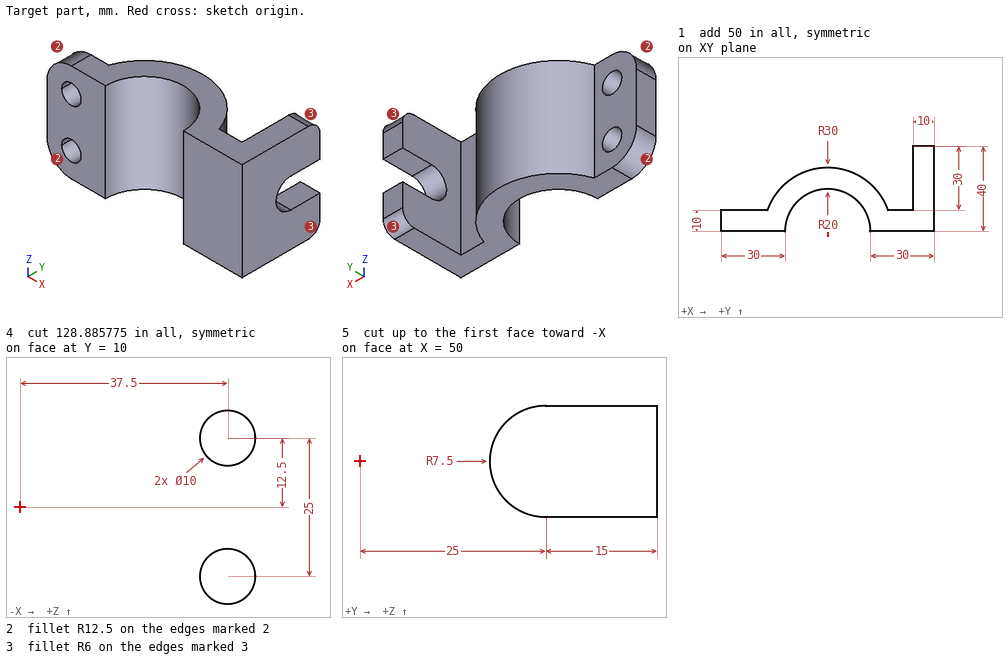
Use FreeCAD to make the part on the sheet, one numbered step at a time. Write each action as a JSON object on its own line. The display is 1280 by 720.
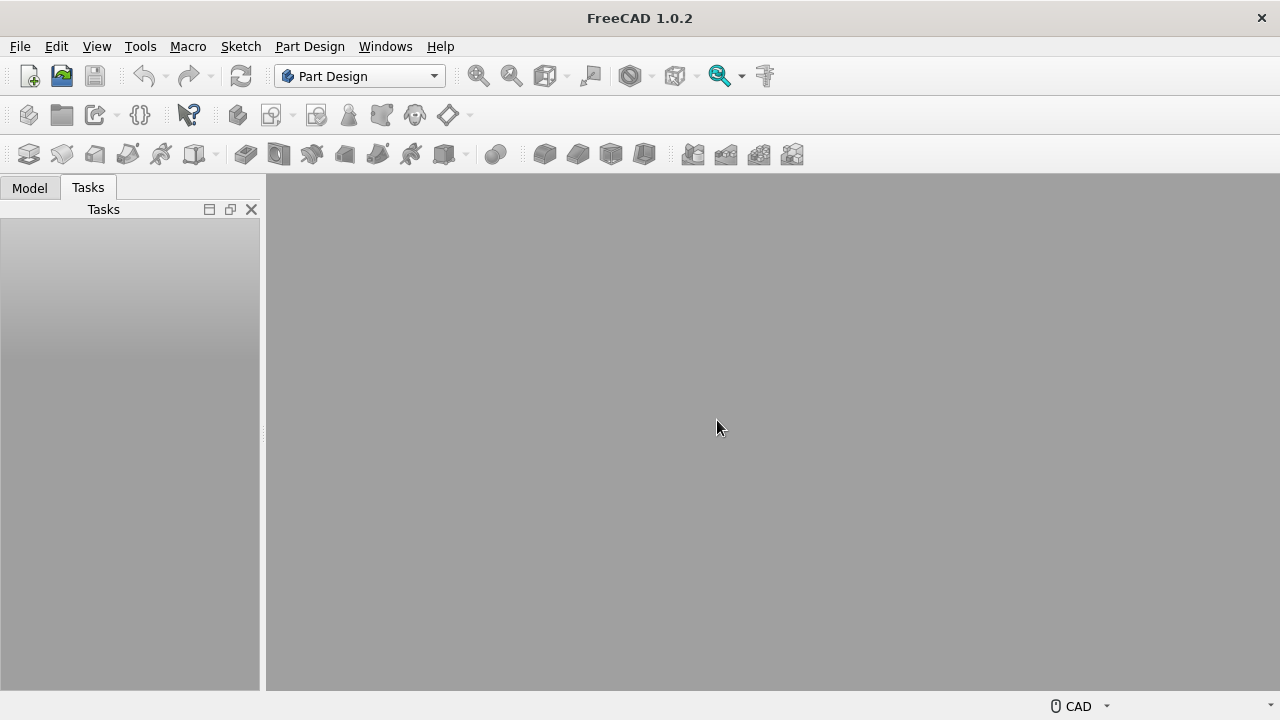
{"action": "left_click", "coordinate": [29, 76]}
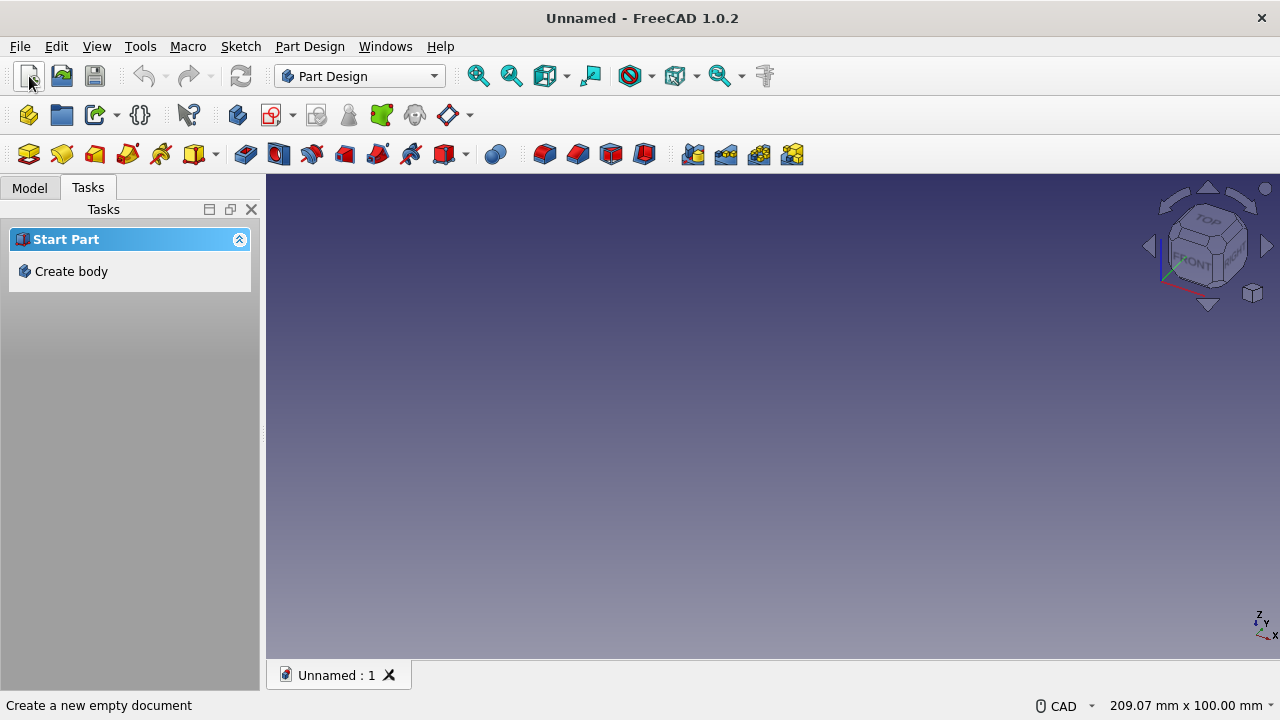
{"action": "left_click", "coordinate": [270, 116]}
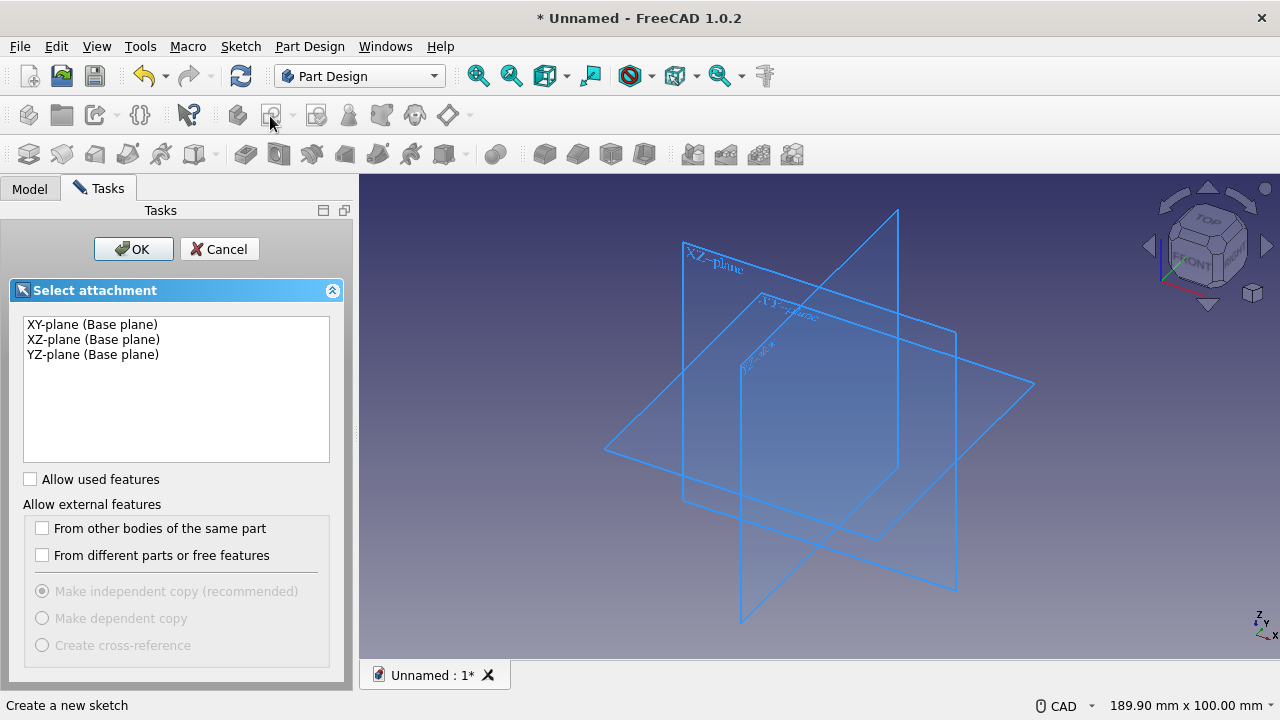
{"action": "left_click", "coordinate": [84, 324]}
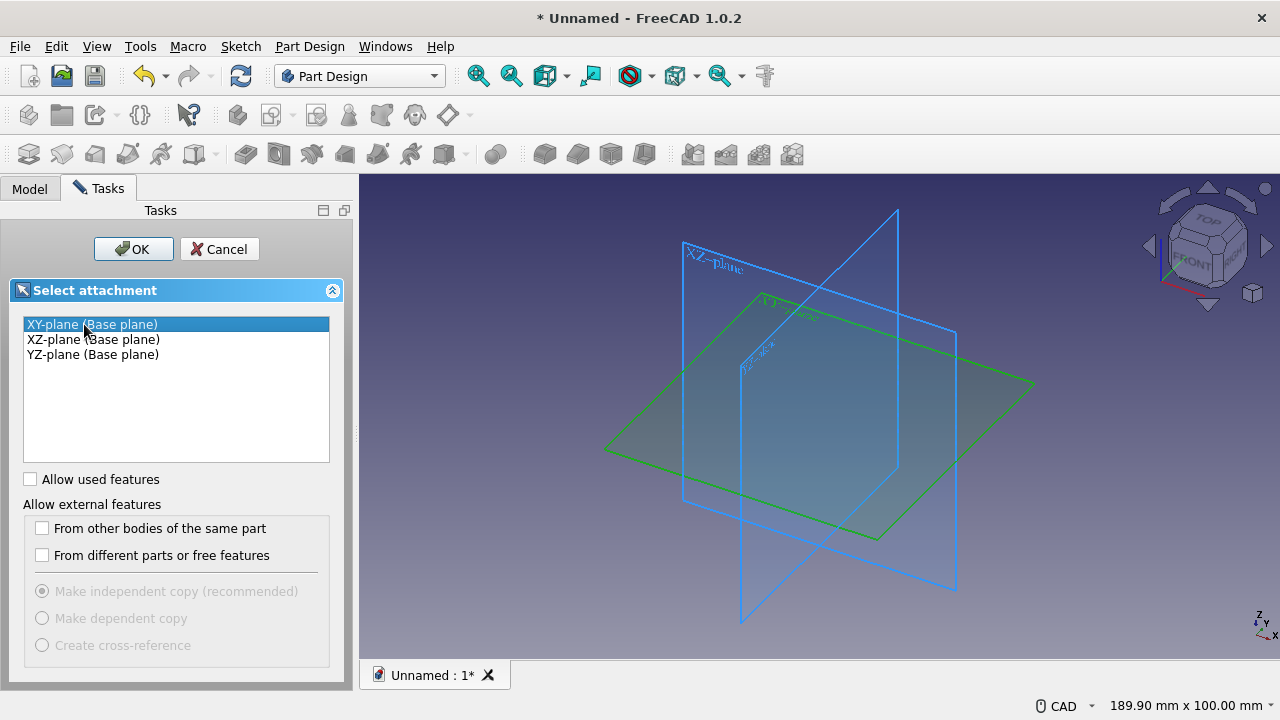
{"action": "left_click", "coordinate": [134, 249]}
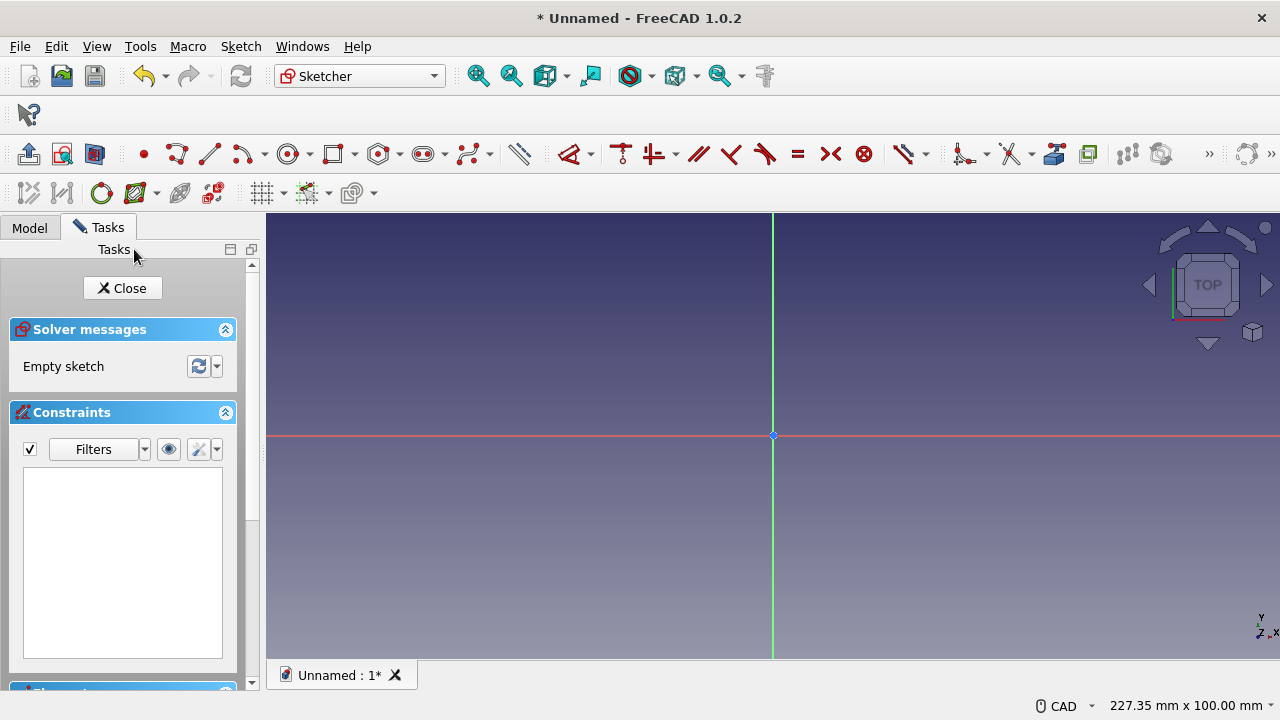
{"action": "scroll", "coordinate": [395, 631], "scroll_direction": "down", "scroll_amount": 1}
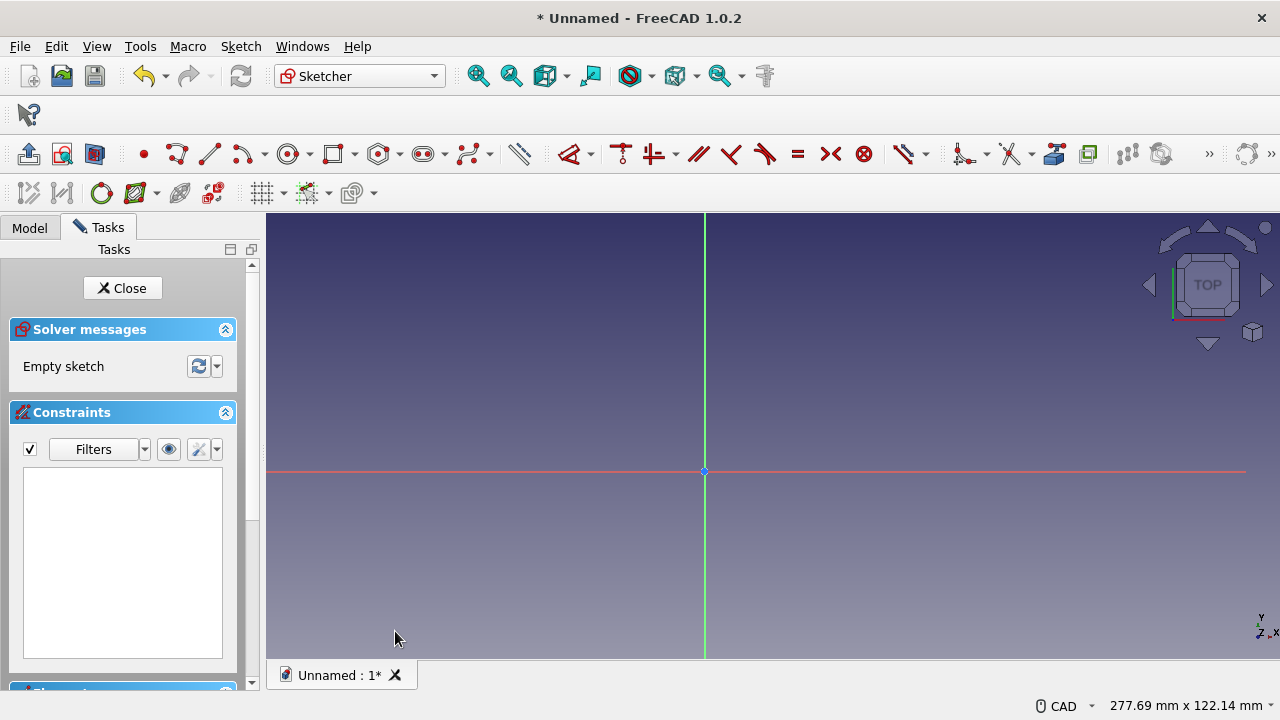
{"action": "scroll", "coordinate": [705, 322], "scroll_direction": "up", "scroll_amount": 2}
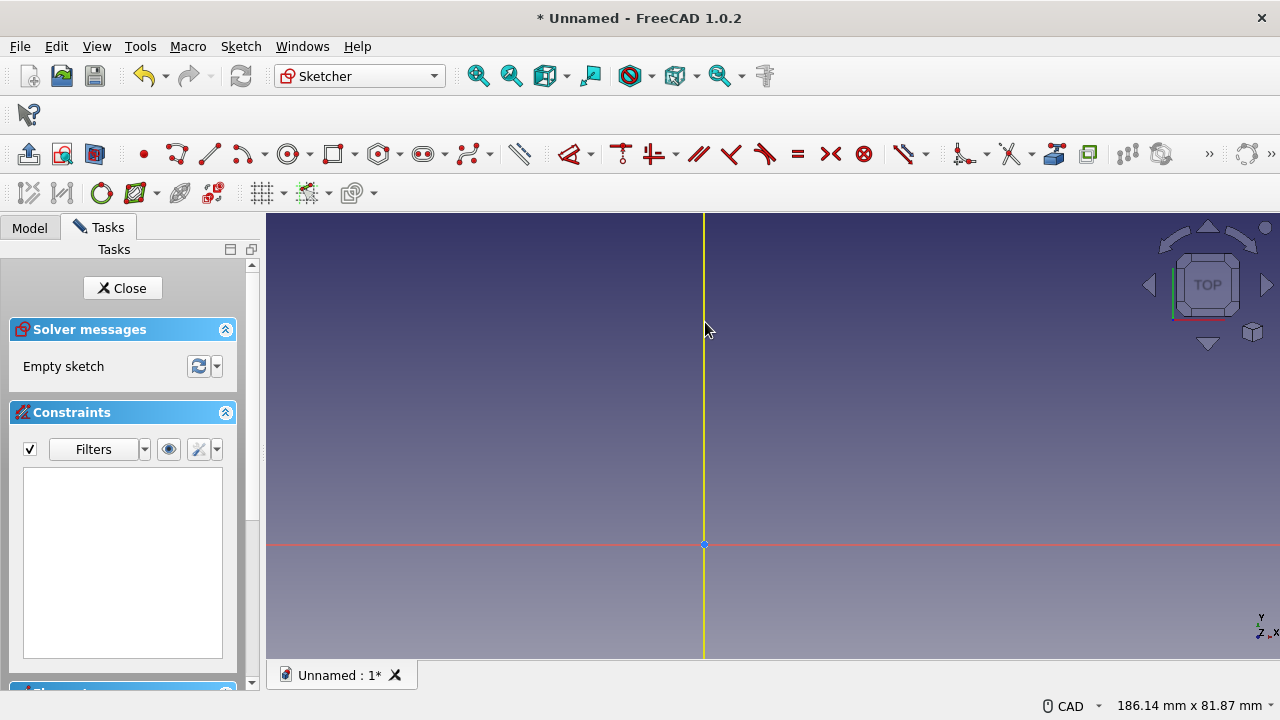
{"action": "left_click", "coordinate": [177, 154]}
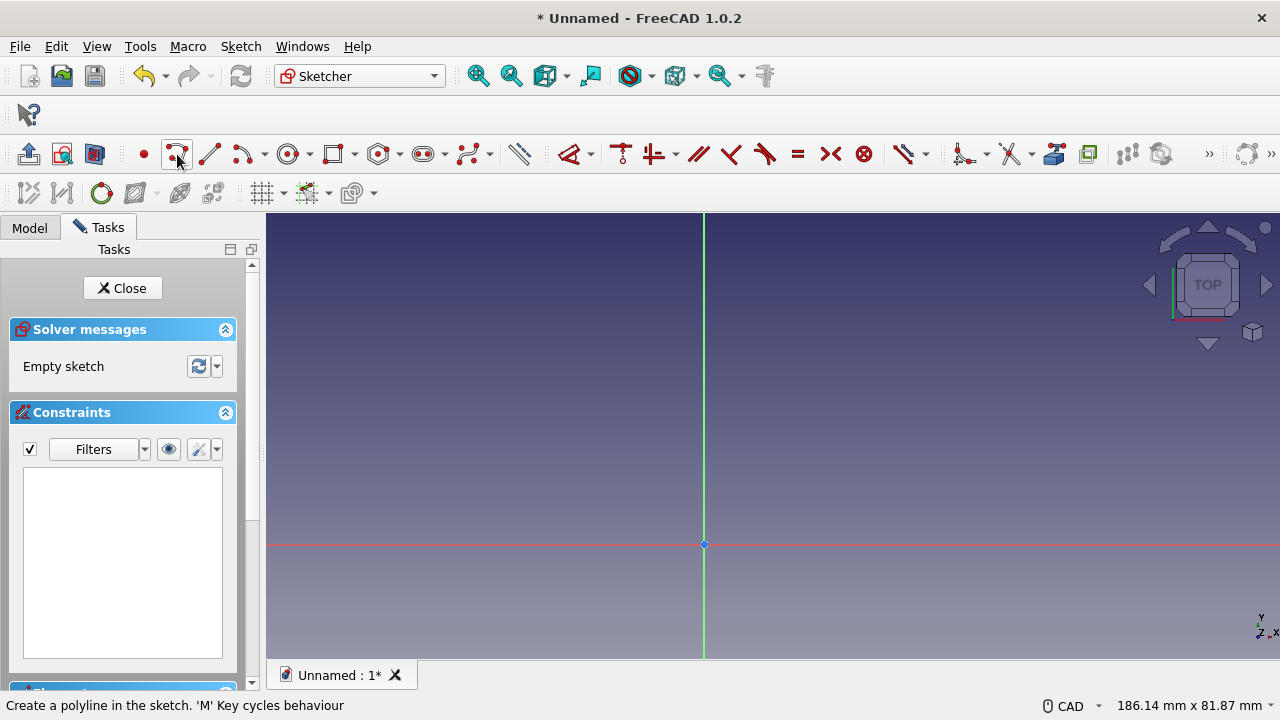
{"action": "left_click", "coordinate": [550, 490]}
{"action": "left_click", "coordinate": [432, 490]}
{"action": "left_click", "coordinate": [432, 545]}
{"action": "left_click", "coordinate": [595, 536]}
{"action": "right_click", "coordinate": [595, 536]}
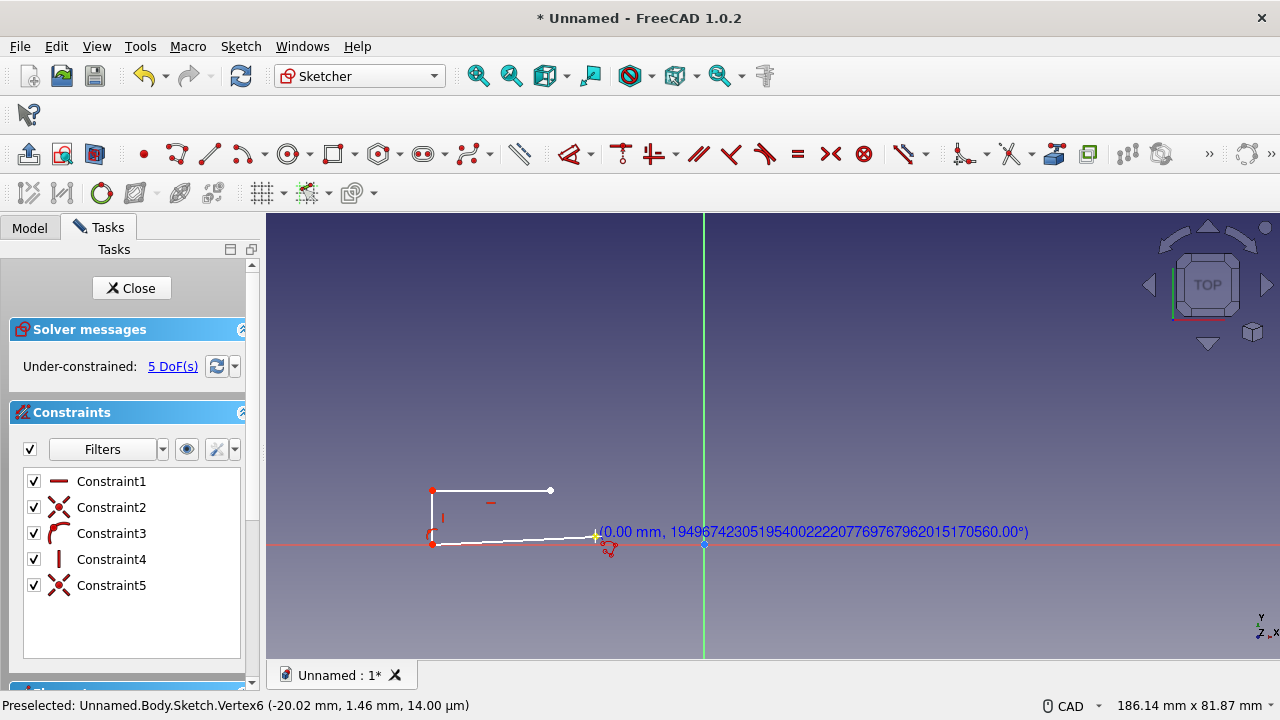
{"action": "left_click", "coordinate": [813, 545]}
{"action": "left_click", "coordinate": [976, 536]}
{"action": "left_click", "coordinate": [976, 327]}
{"action": "left_click", "coordinate": [922, 327]}
{"action": "left_click", "coordinate": [922, 490]}
{"action": "left_click", "coordinate": [858, 490]}
{"action": "right_click", "coordinate": [858, 490]}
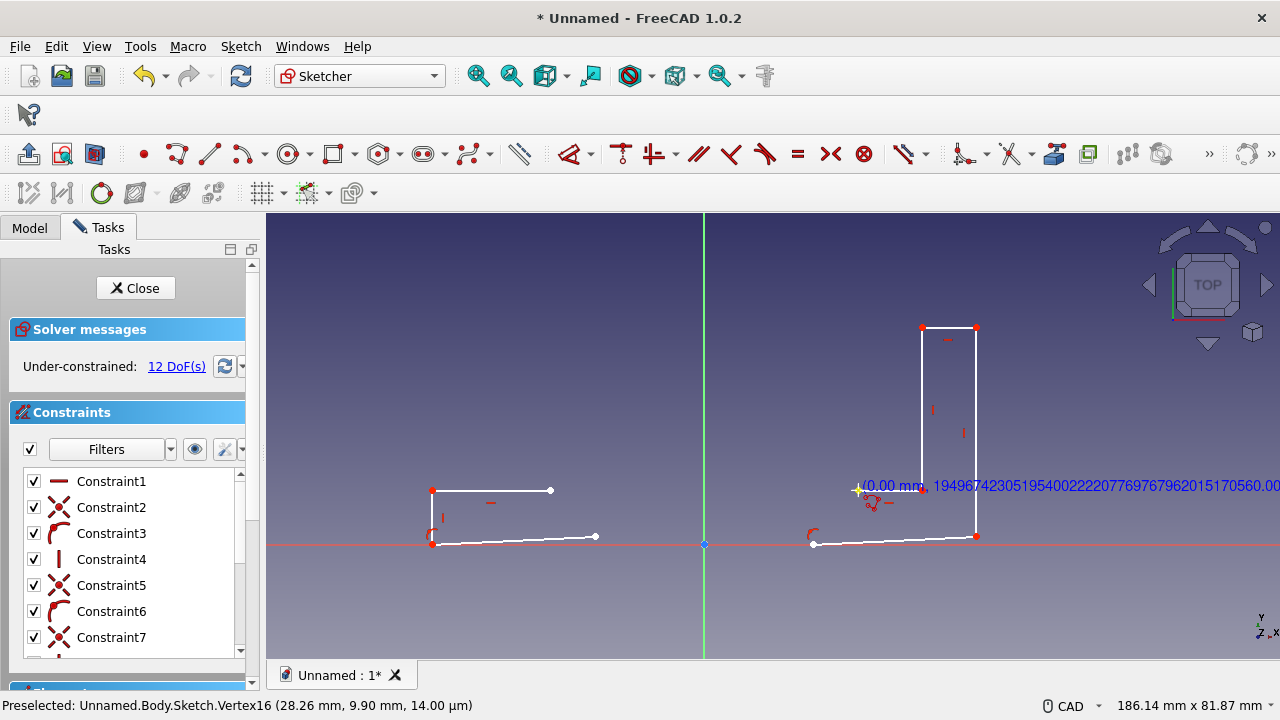
{"action": "key", "text": "g 3 a"}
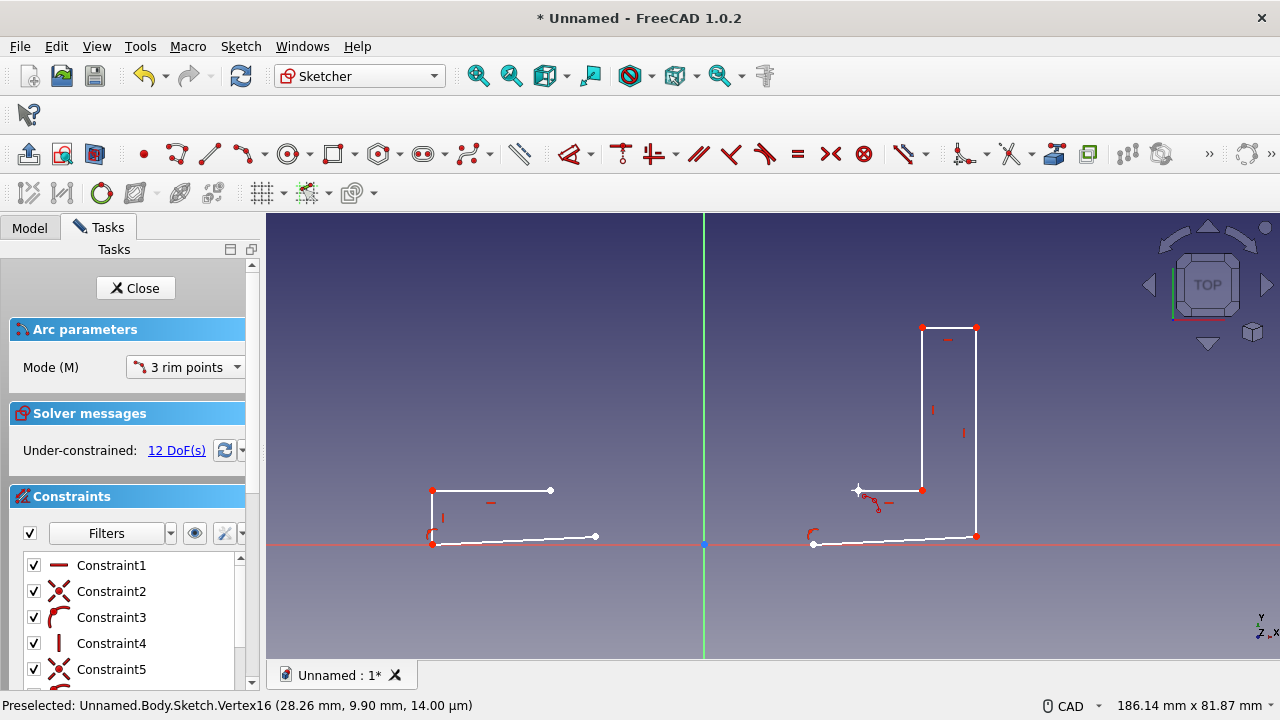
{"action": "left_click", "coordinate": [595, 537]}
{"action": "left_click", "coordinate": [813, 545]}
{"action": "left_click", "coordinate": [738, 441]}